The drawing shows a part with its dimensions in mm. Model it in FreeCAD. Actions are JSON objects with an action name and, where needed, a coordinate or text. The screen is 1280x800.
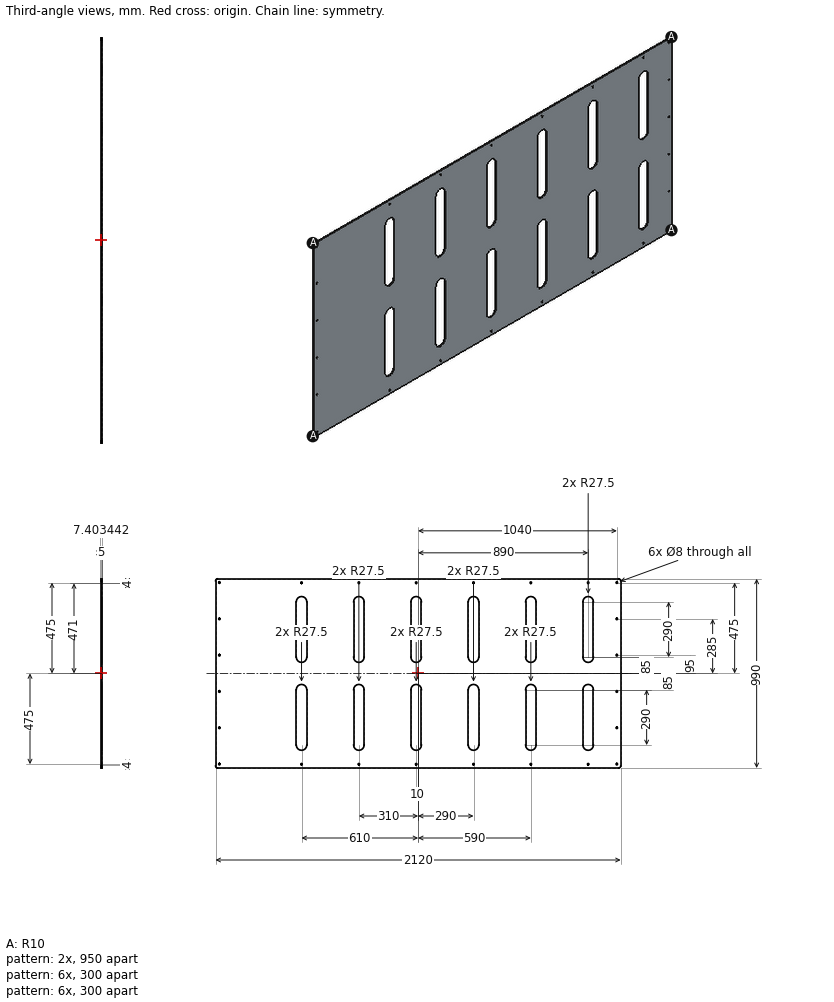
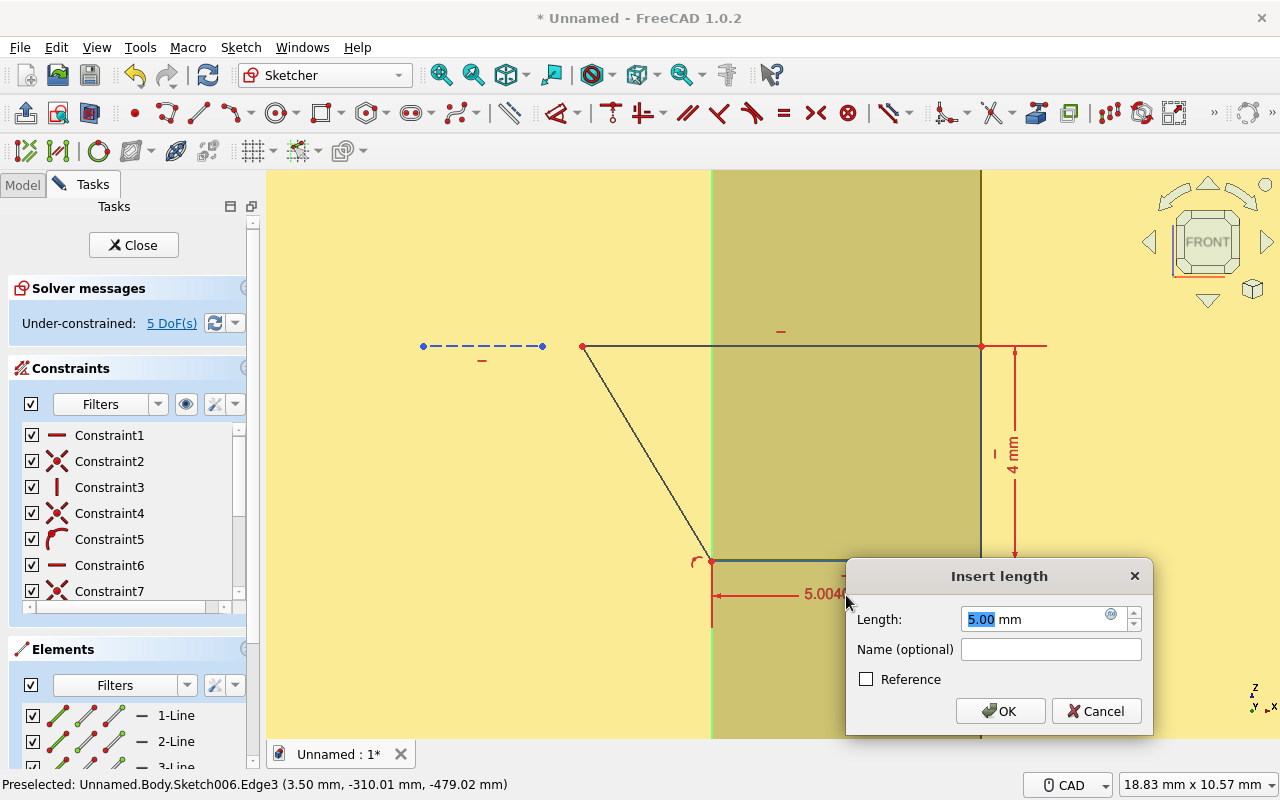
{"action": "type", "text": "5"}
{"action": "key", "text": "Return"}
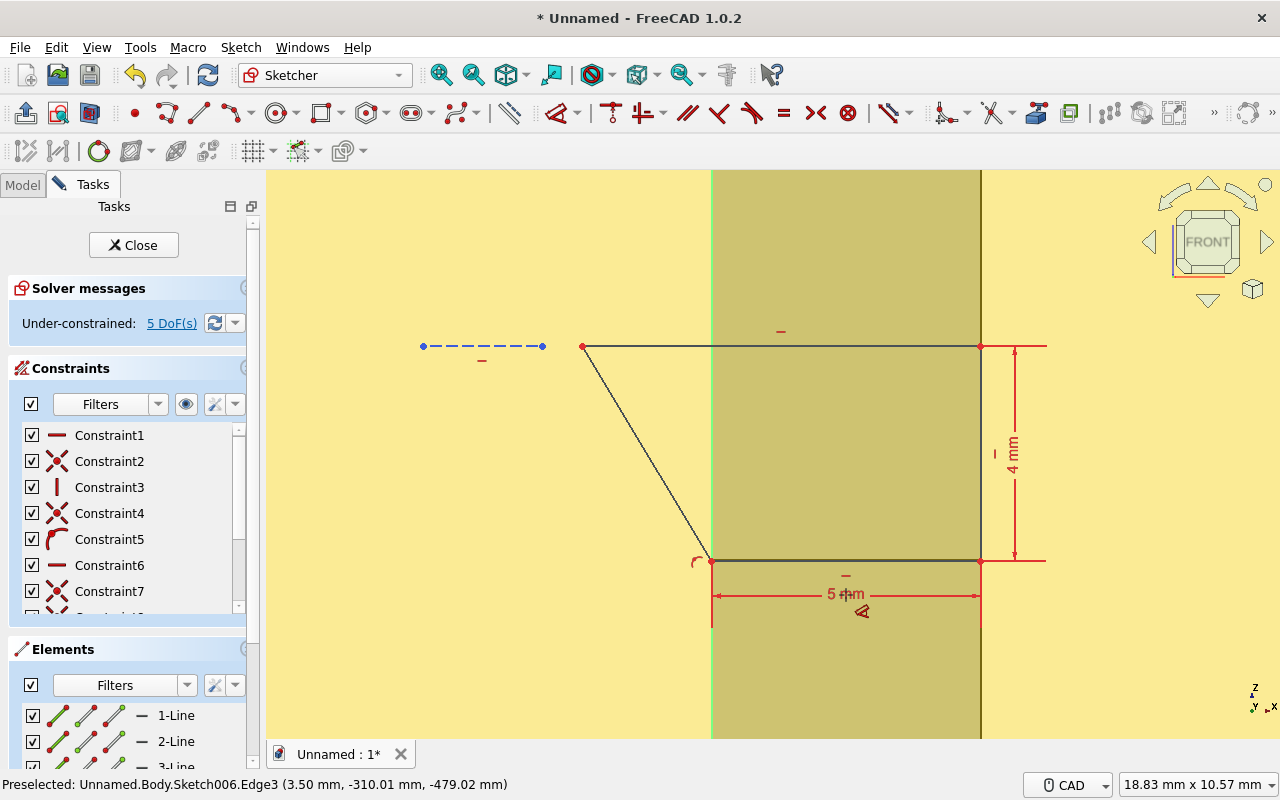
{"action": "left_click", "coordinate": [582, 346]}
{"action": "left_click", "coordinate": [548, 272]}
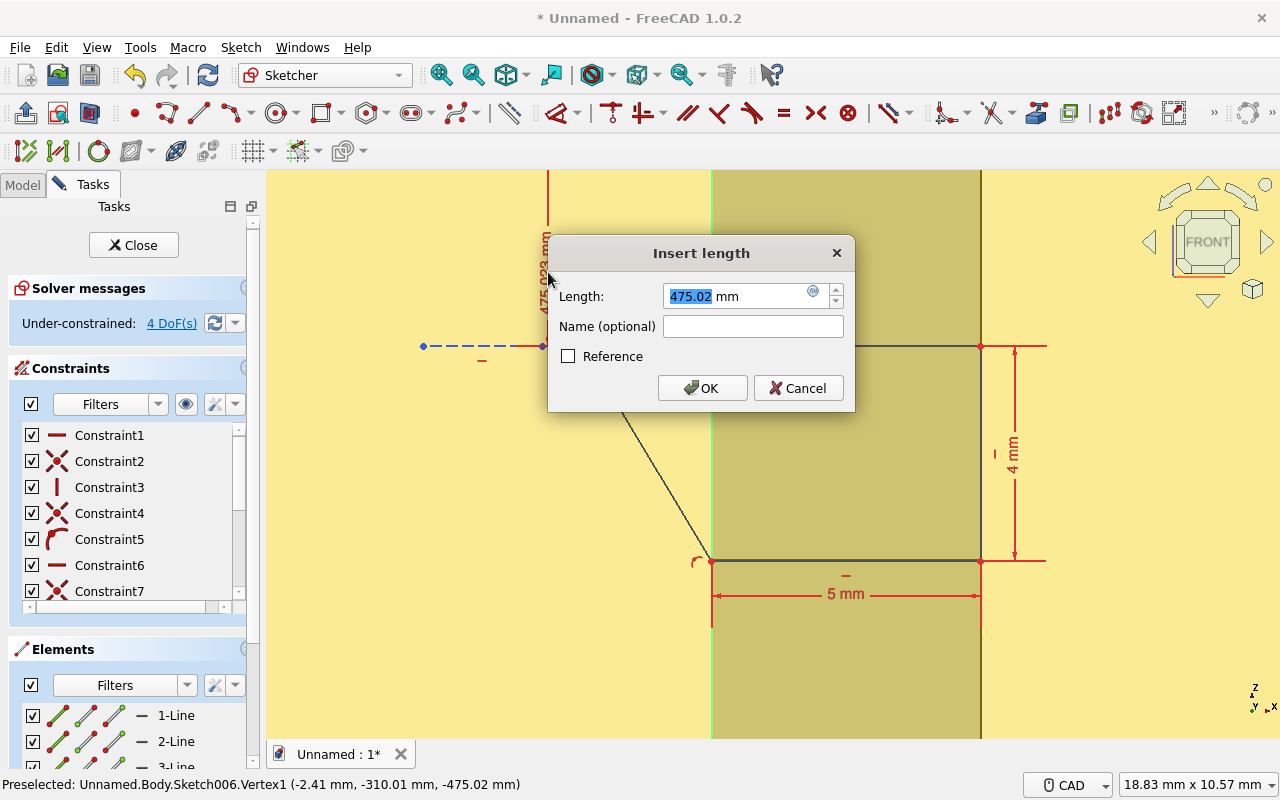
{"action": "type", "text": "475"}
{"action": "key", "text": "Return"}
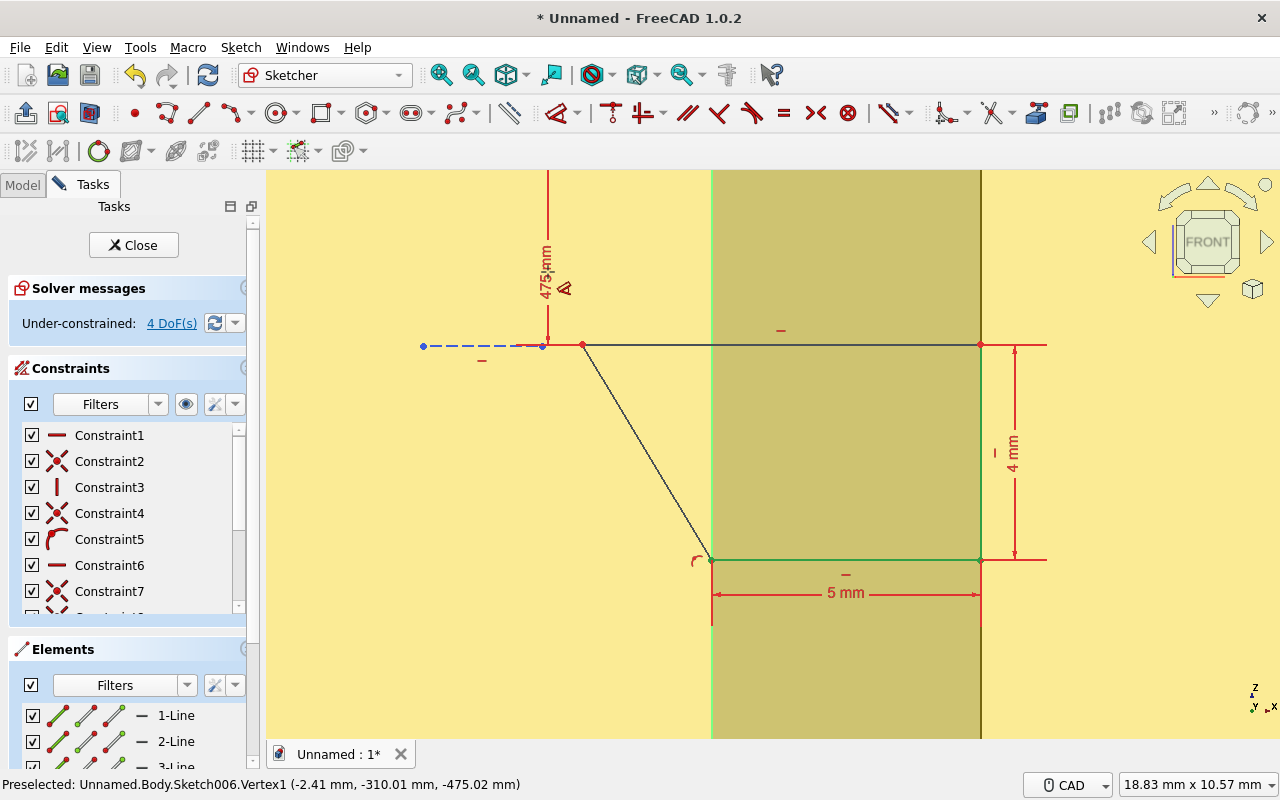
{"action": "left_click", "coordinate": [542, 346]}
{"action": "left_click", "coordinate": [508, 238]}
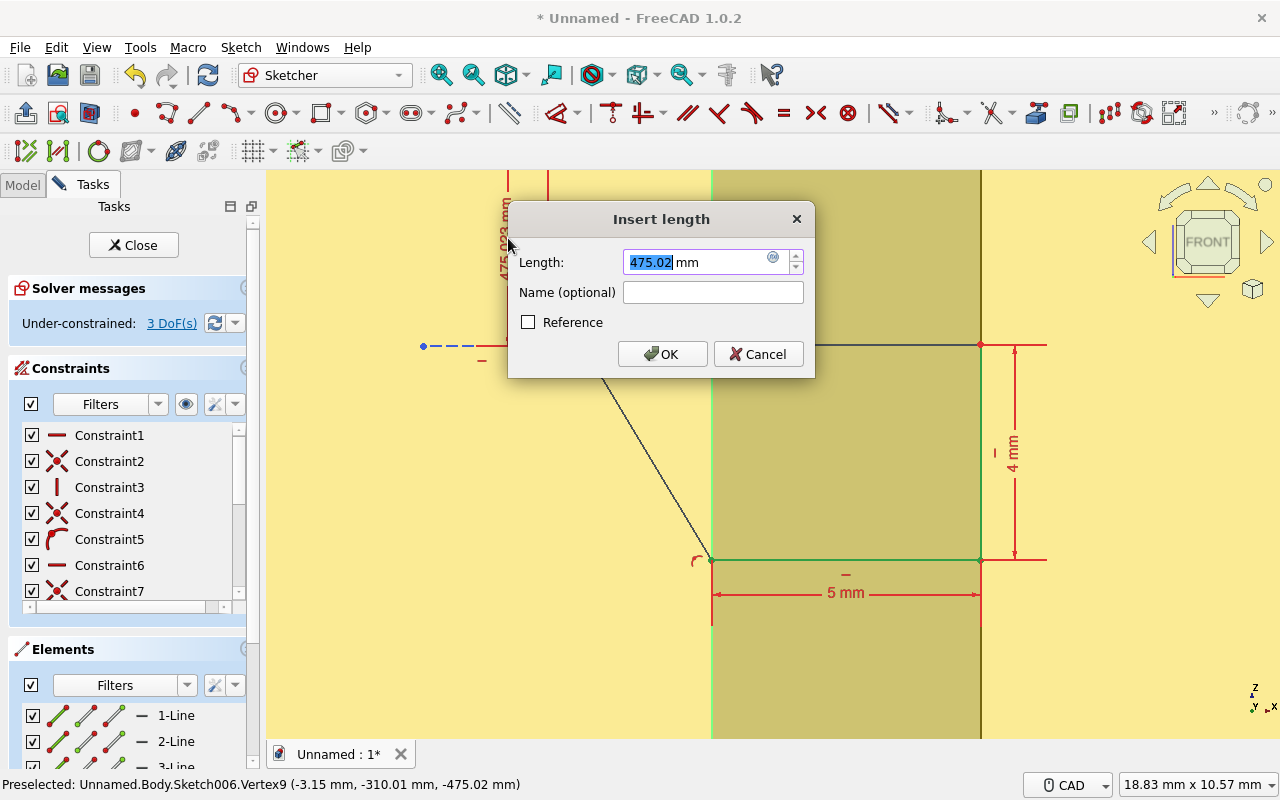
{"action": "type", "text": "475"}
{"action": "key", "text": "Return"}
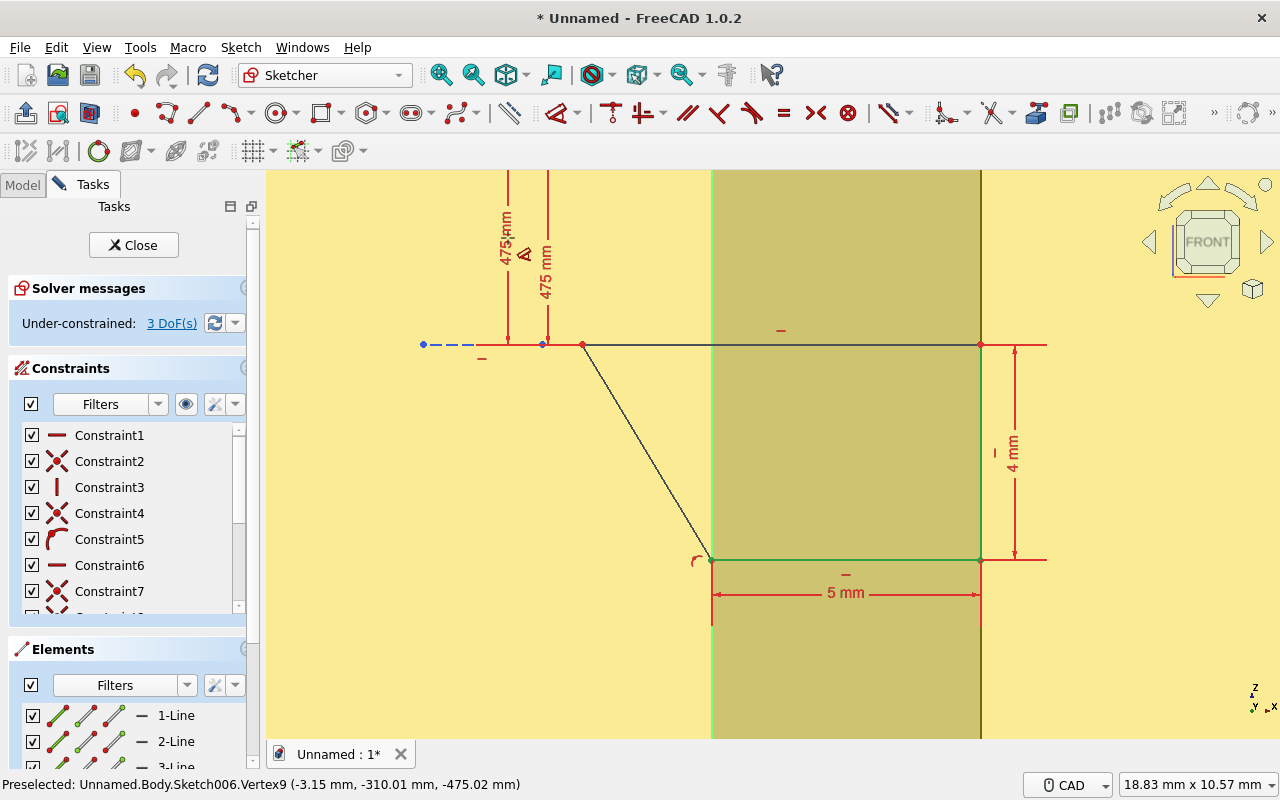
{"action": "scroll", "coordinate": [702, 345], "scroll_direction": "up", "scroll_amount": 2}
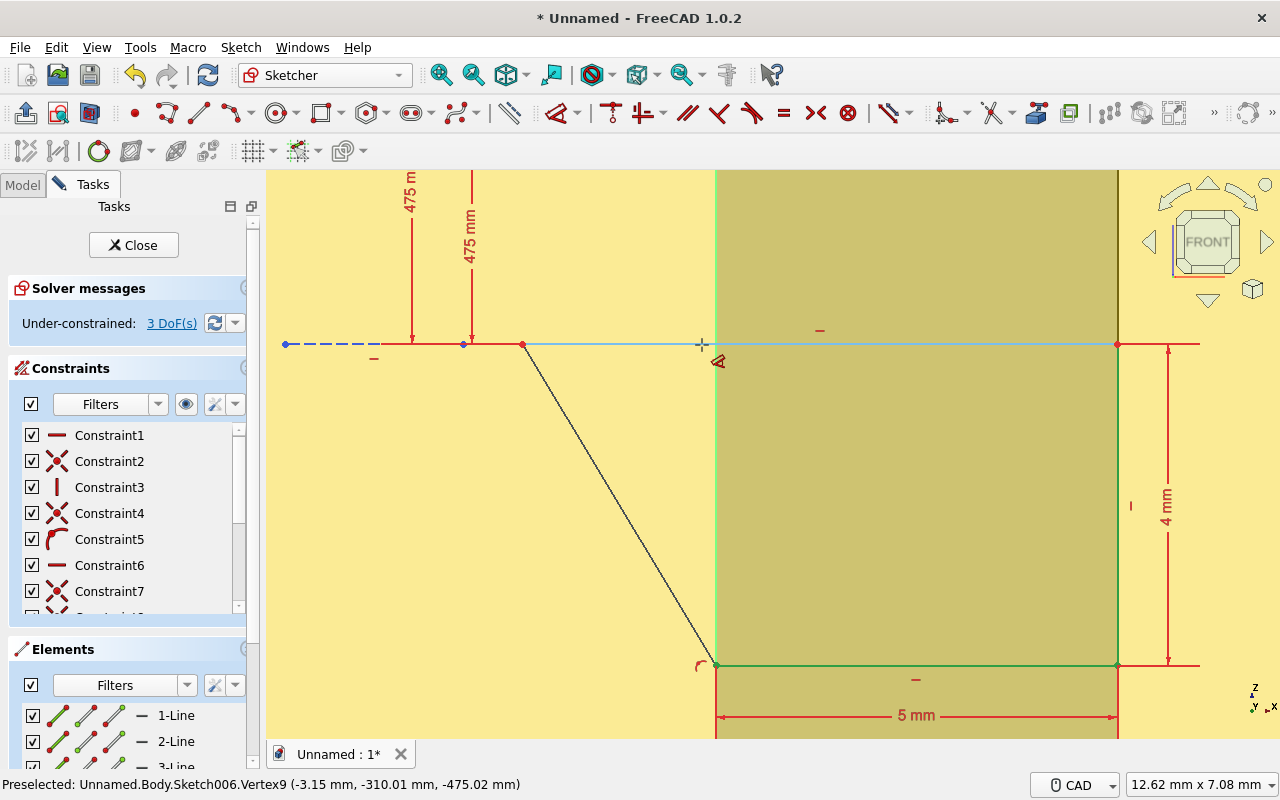
{"action": "left_click", "coordinate": [701, 344]}
{"action": "left_click", "coordinate": [819, 310]}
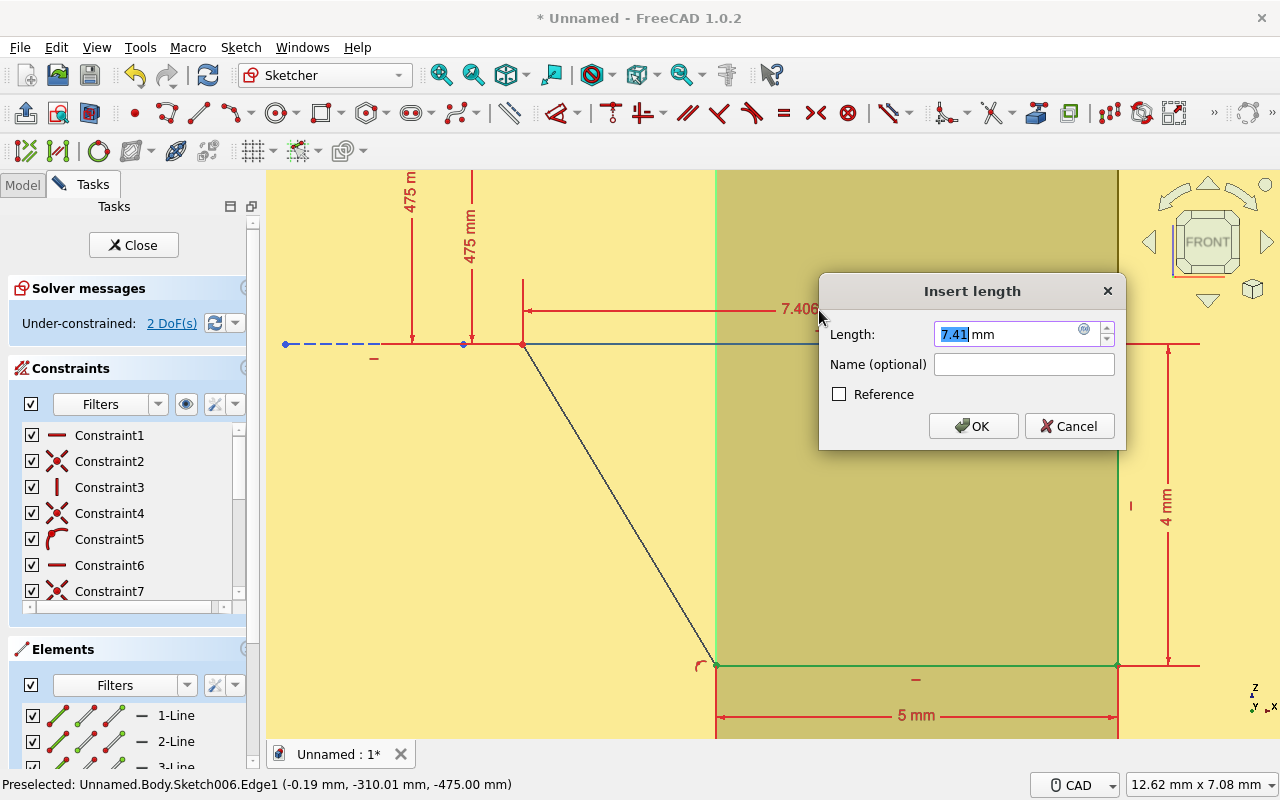
{"action": "type", "text": "7.403442"}
{"action": "key", "text": "Return"}
{"action": "key", "text": "Escape"}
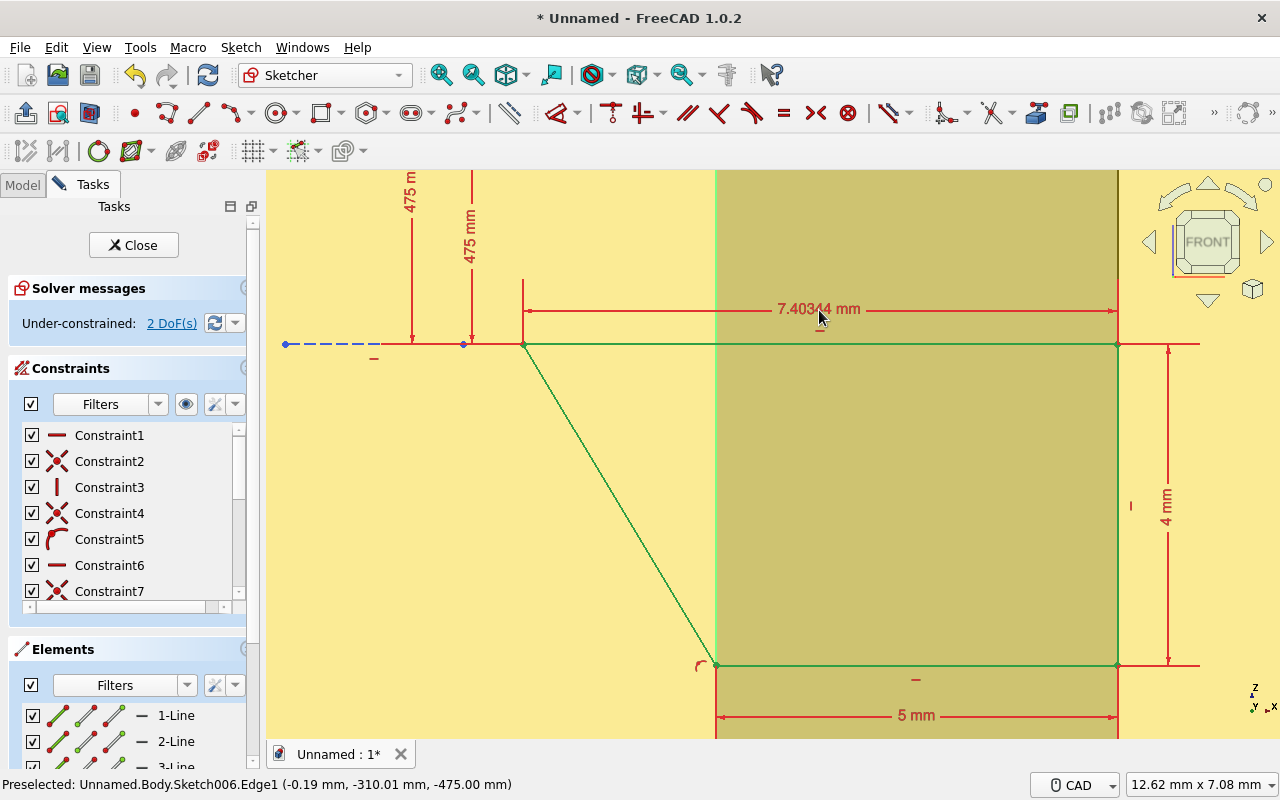
{"action": "left_click", "coordinate": [134, 245]}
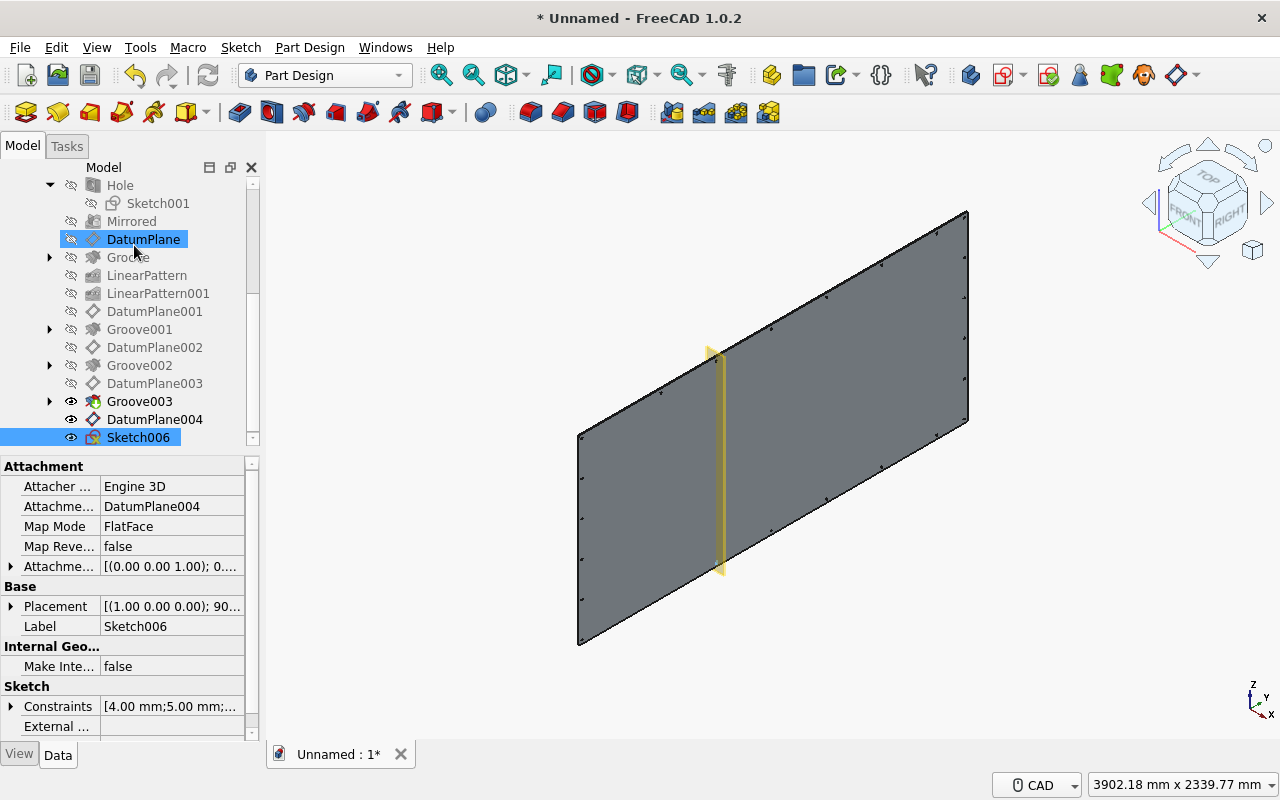
{"action": "left_click", "coordinate": [304, 112]}